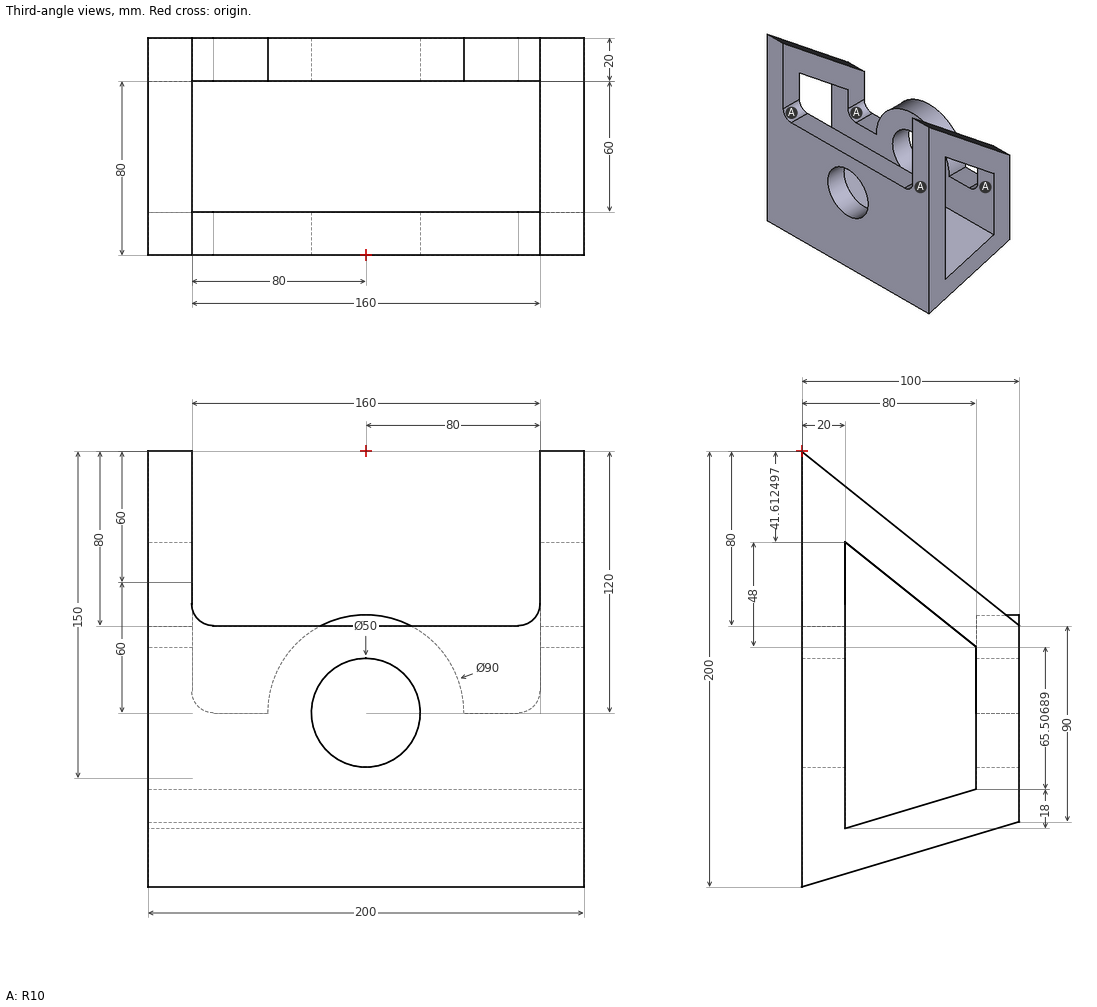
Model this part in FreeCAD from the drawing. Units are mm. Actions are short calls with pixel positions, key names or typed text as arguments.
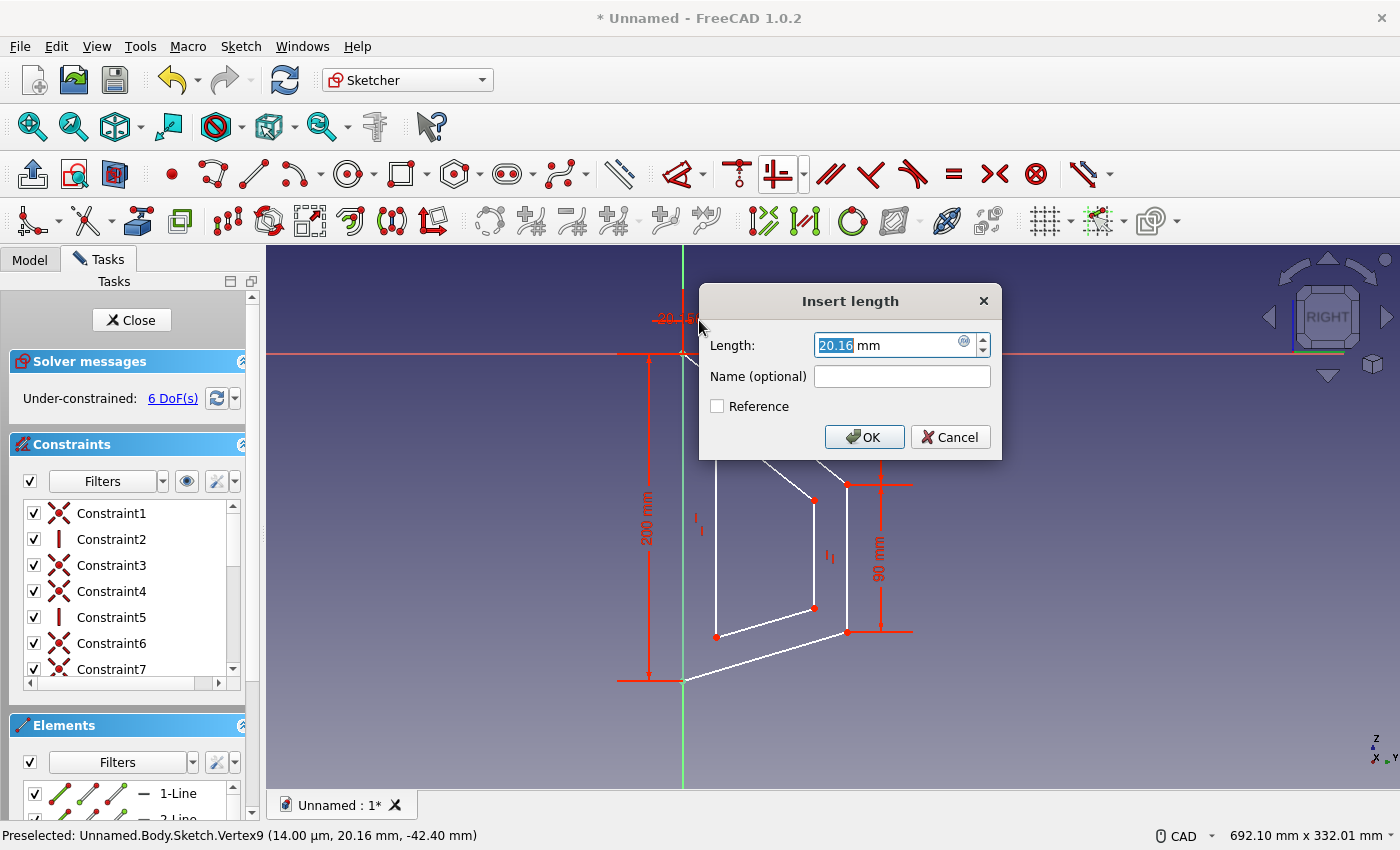
text(20)
key(Return)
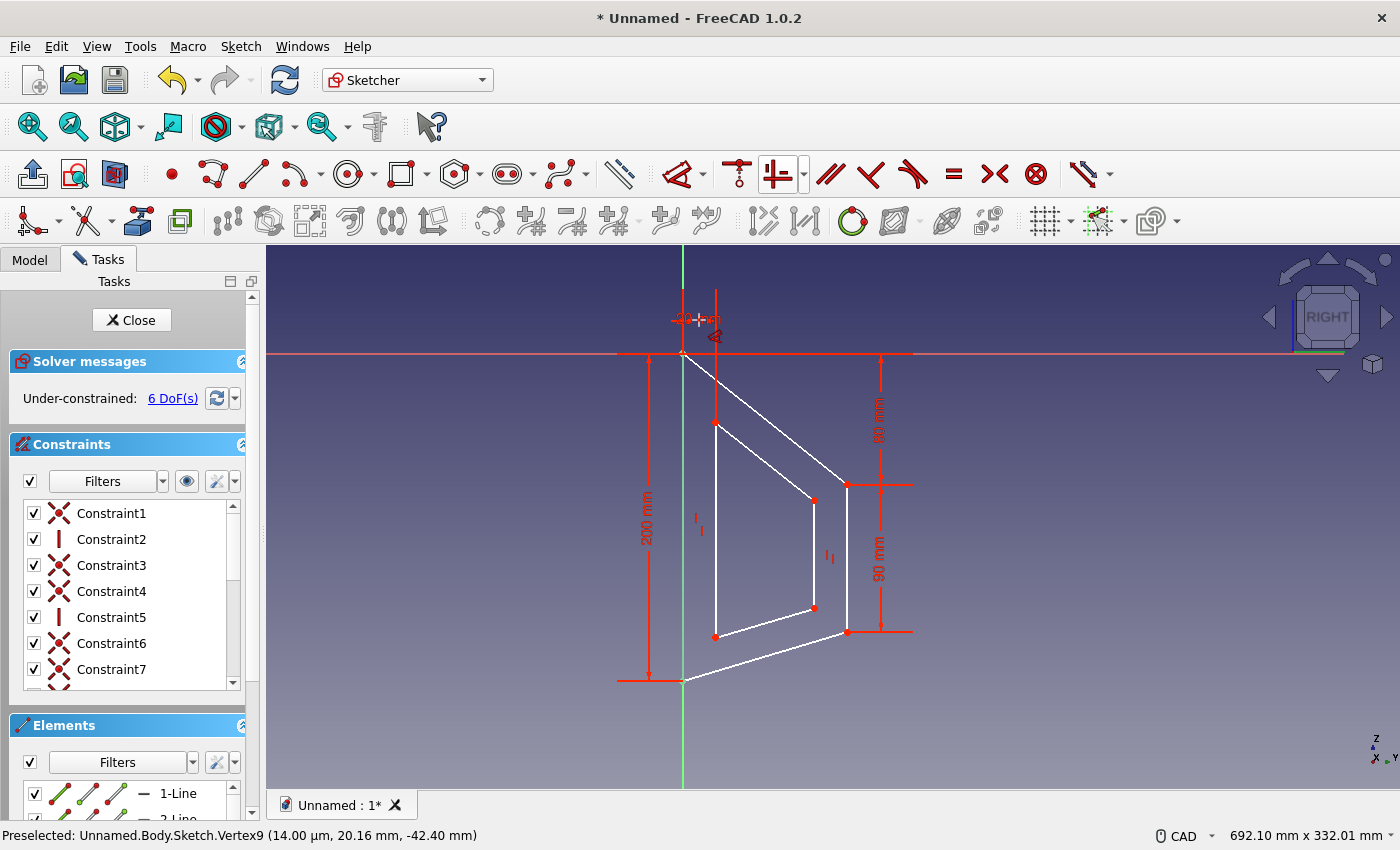
click(814, 501)
click(779, 320)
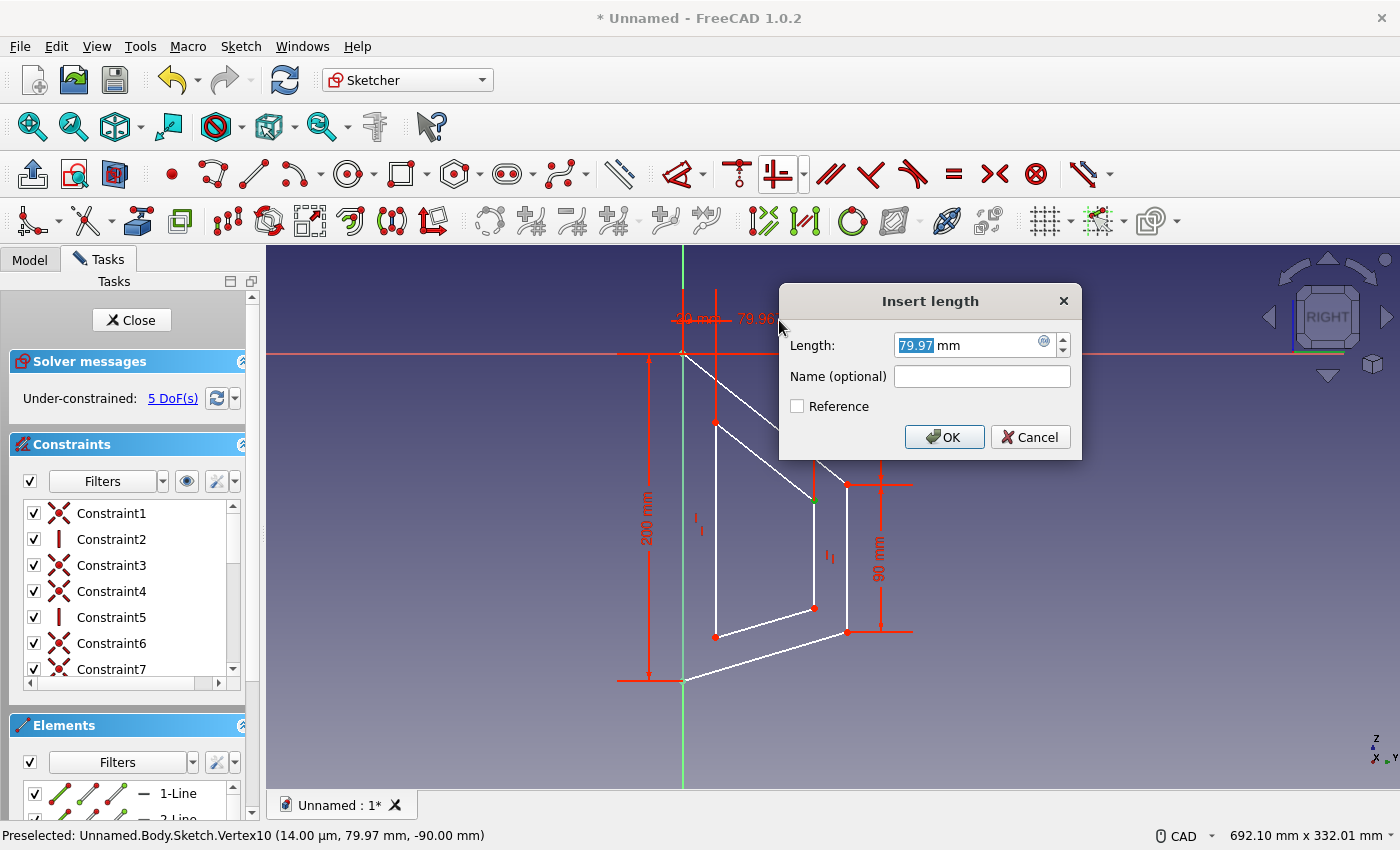
text(80)
key(Return)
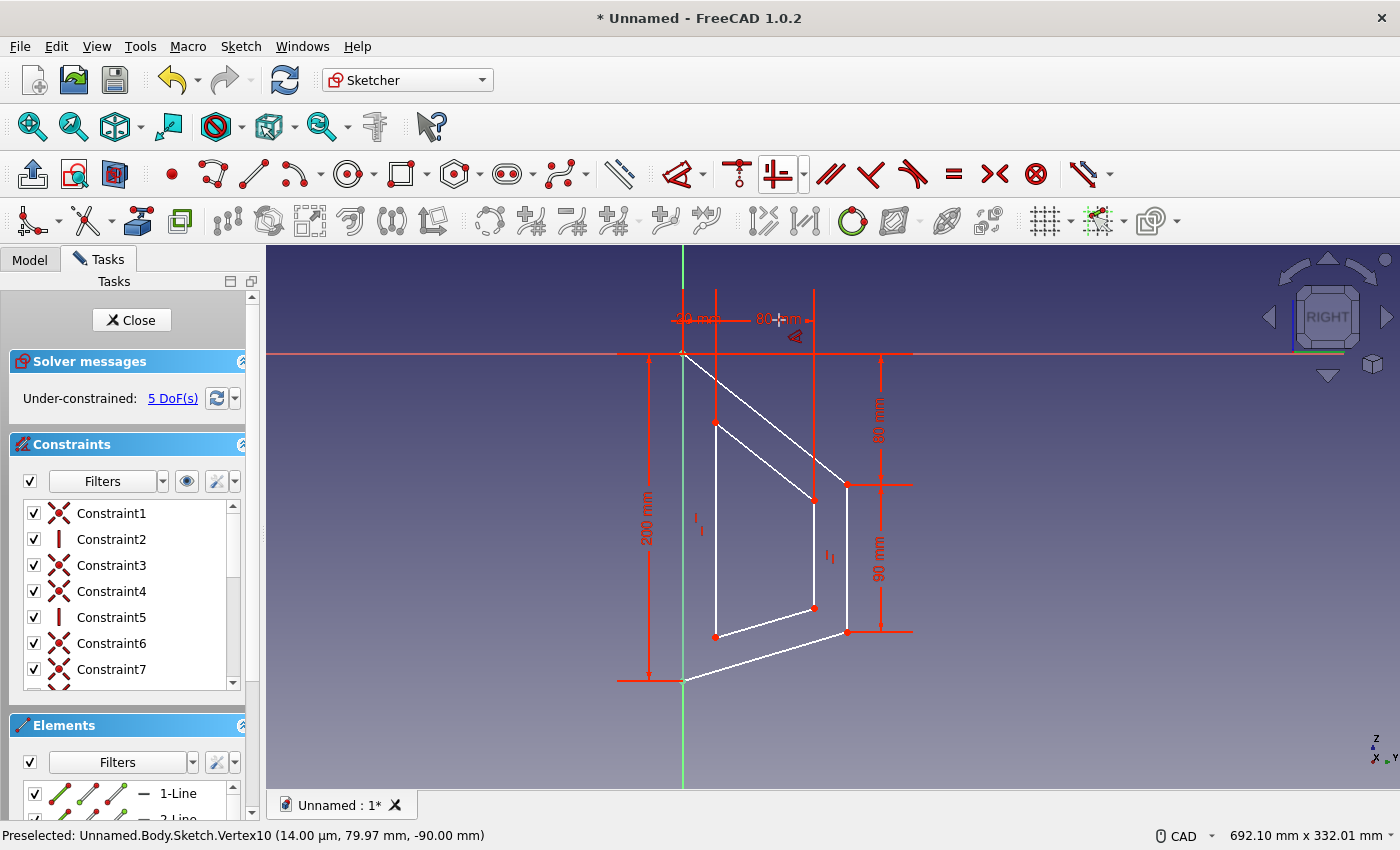
click(745, 446)
click(848, 462)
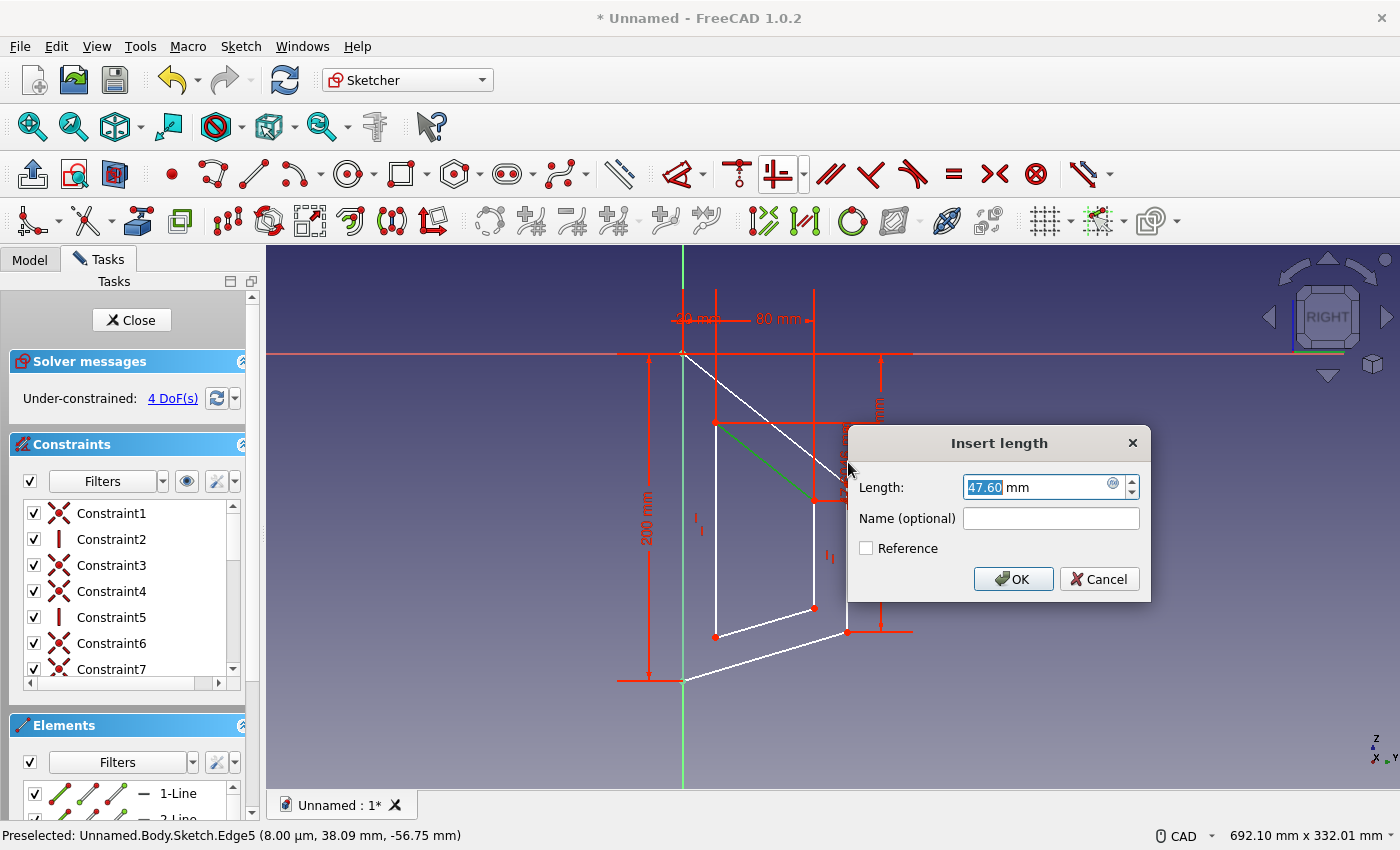
text(48)
key(Return)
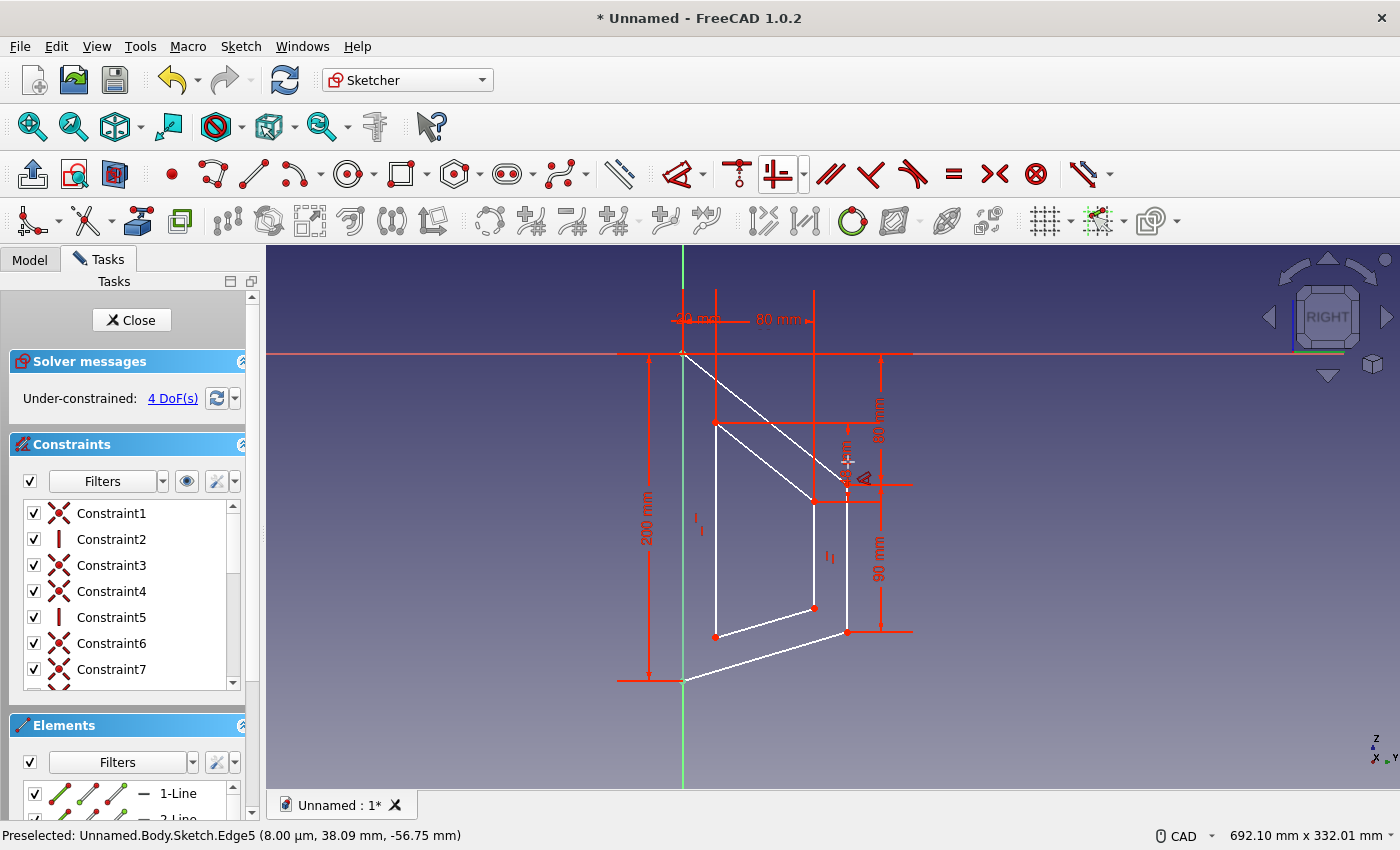
scroll(785, 618, up, 2)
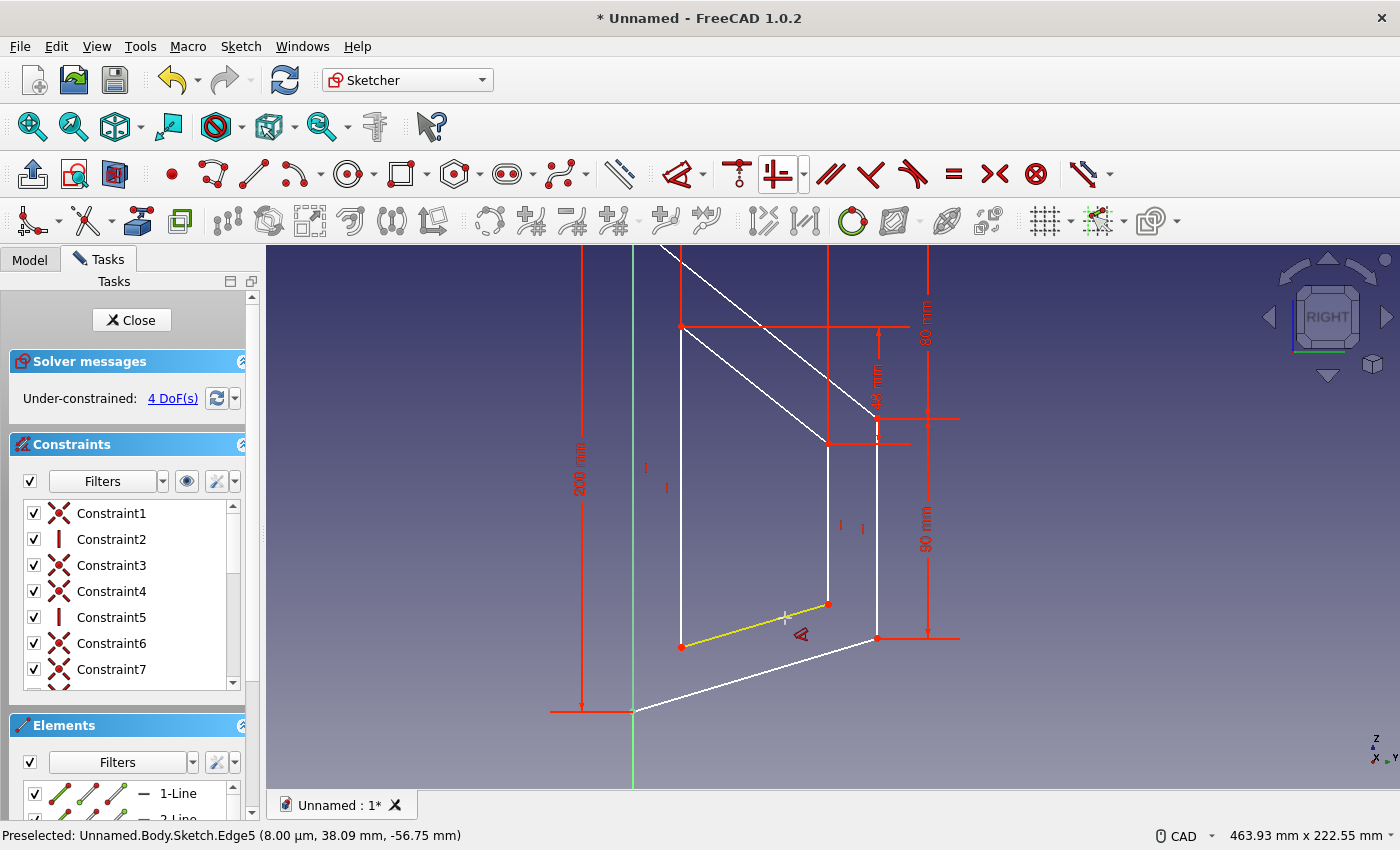
click(784, 617)
click(862, 626)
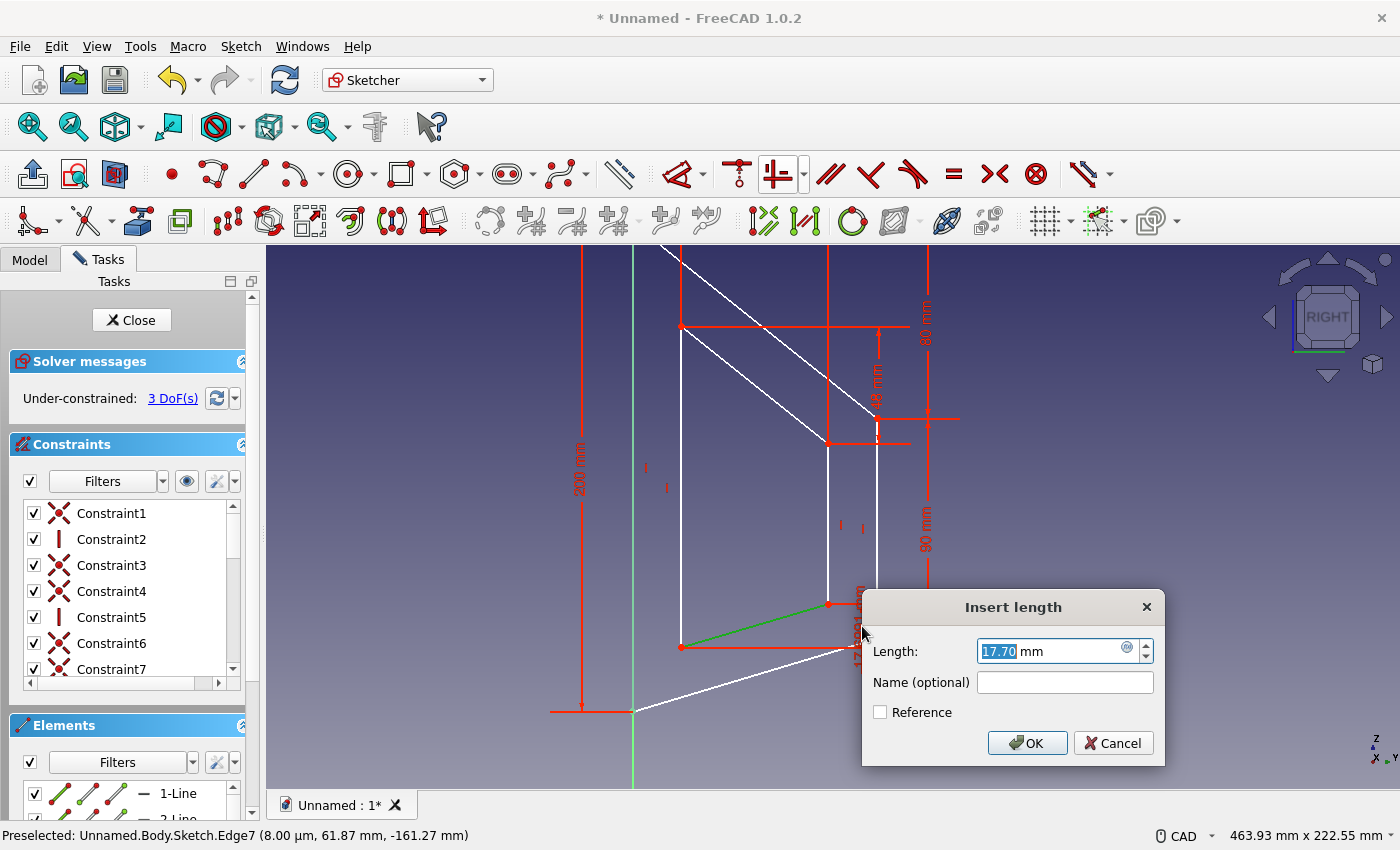
text(18)
key(Return)